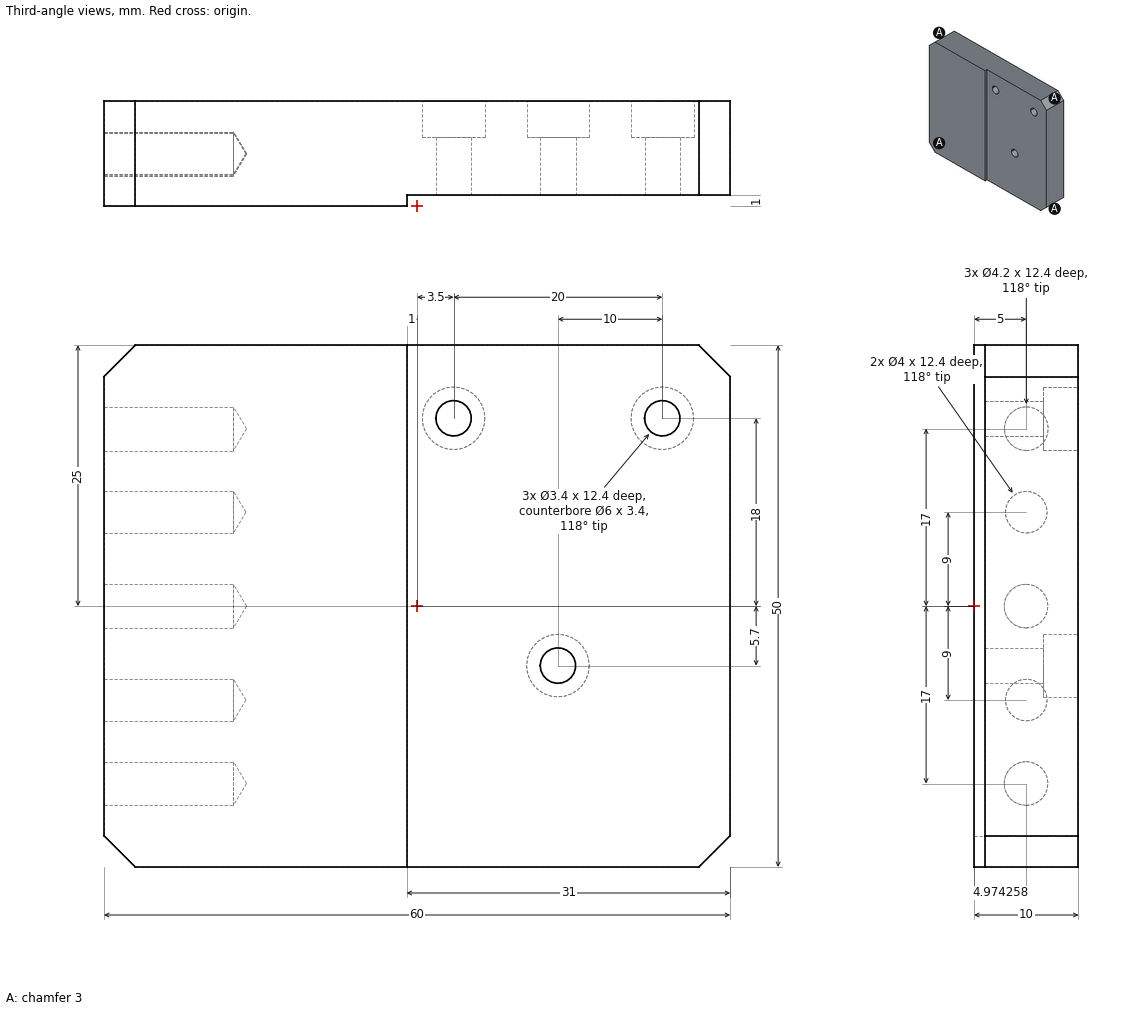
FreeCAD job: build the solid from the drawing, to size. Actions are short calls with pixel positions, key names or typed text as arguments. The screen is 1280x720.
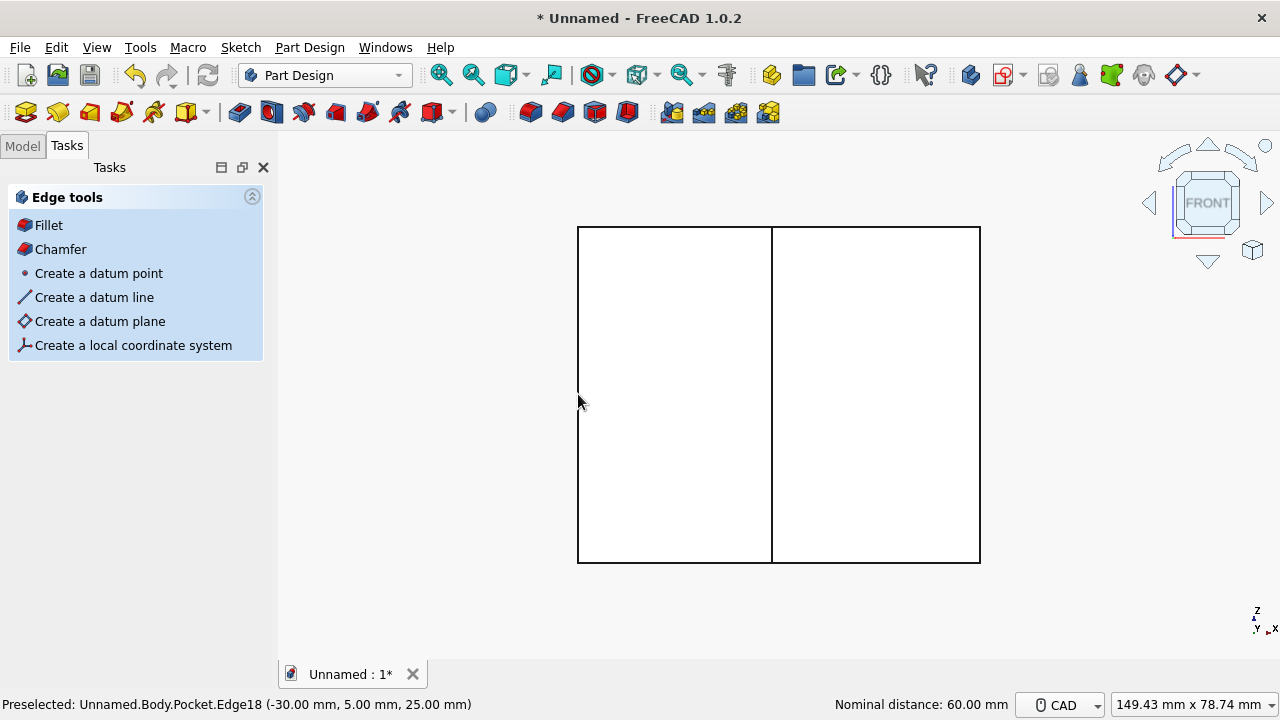
key(3)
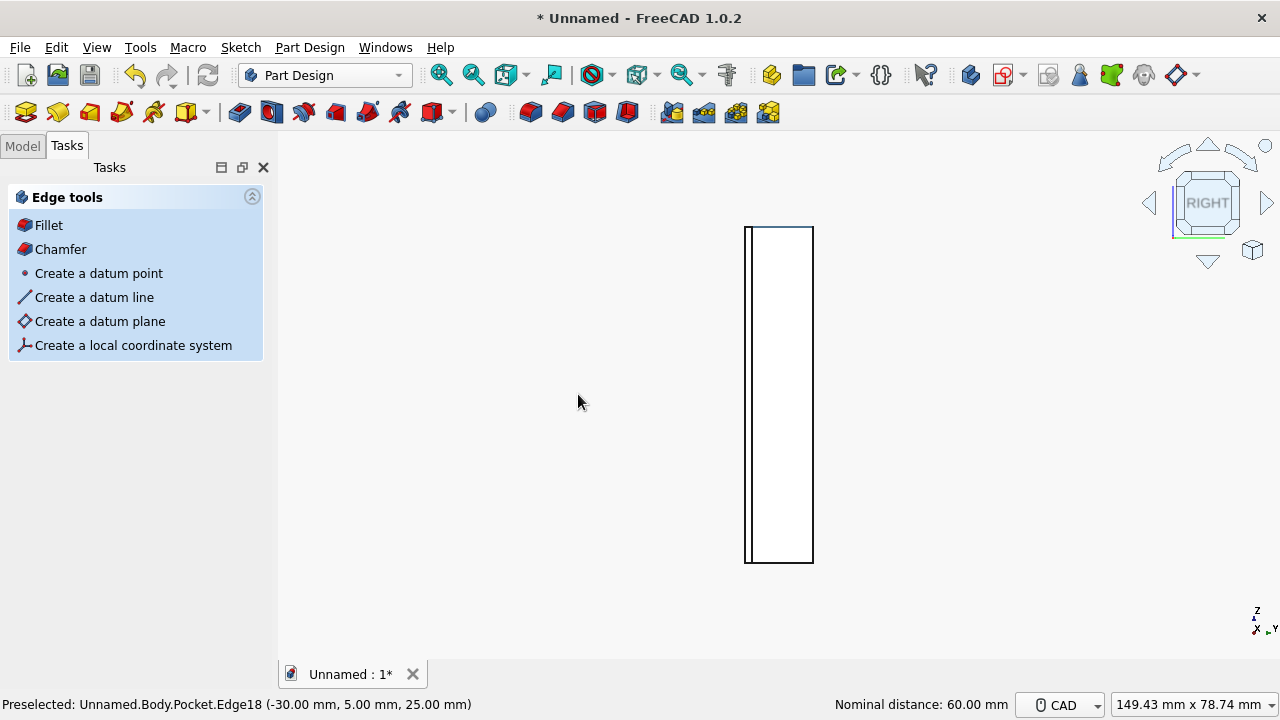
click(782, 562, ctrl)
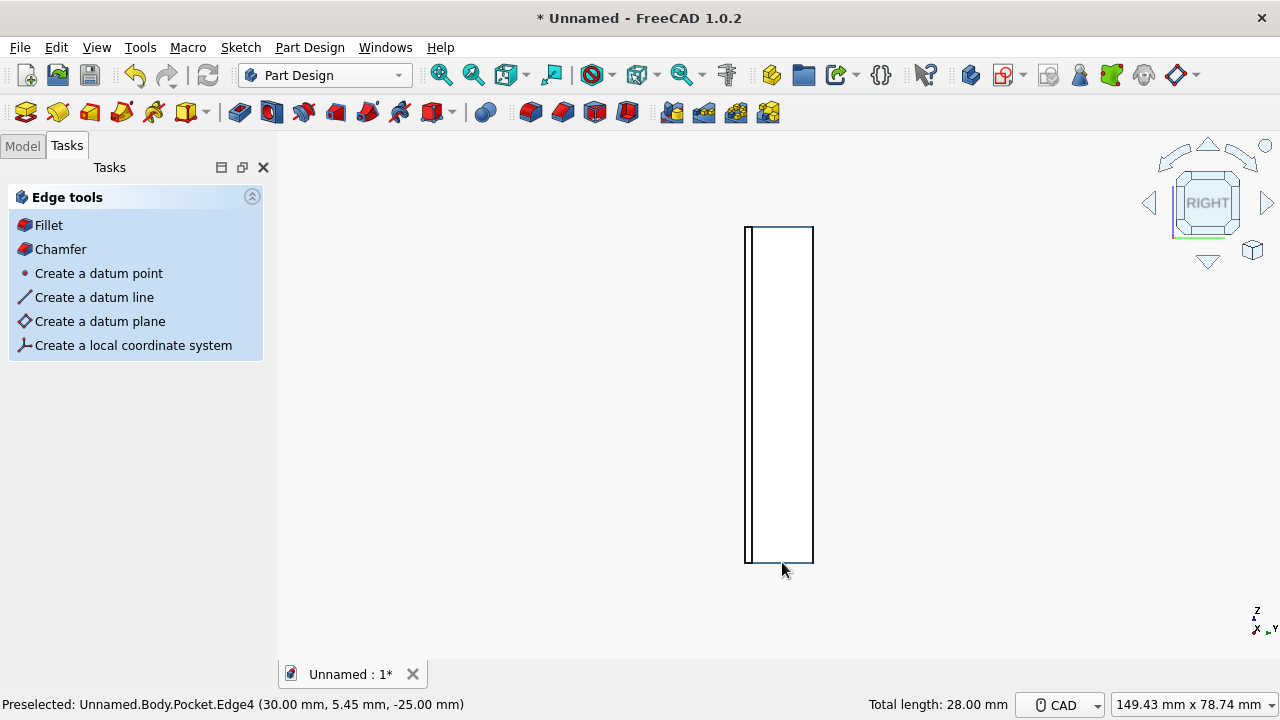
key(5)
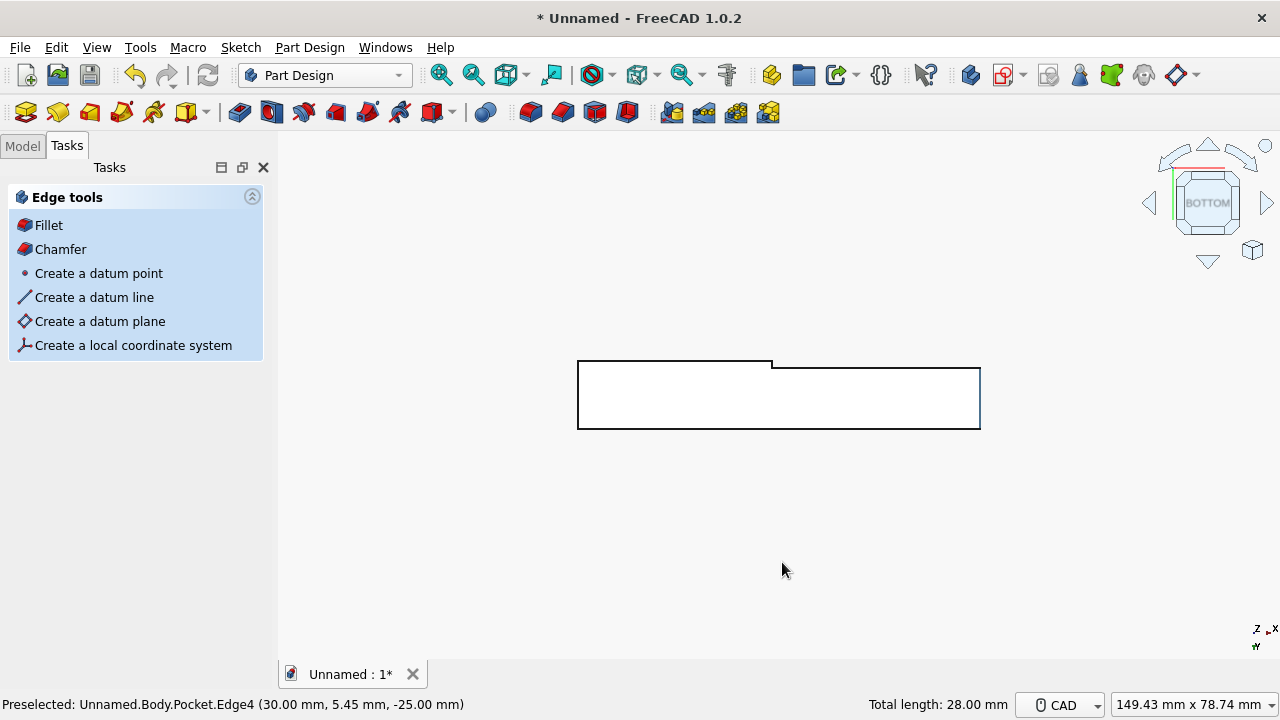
click(442, 76)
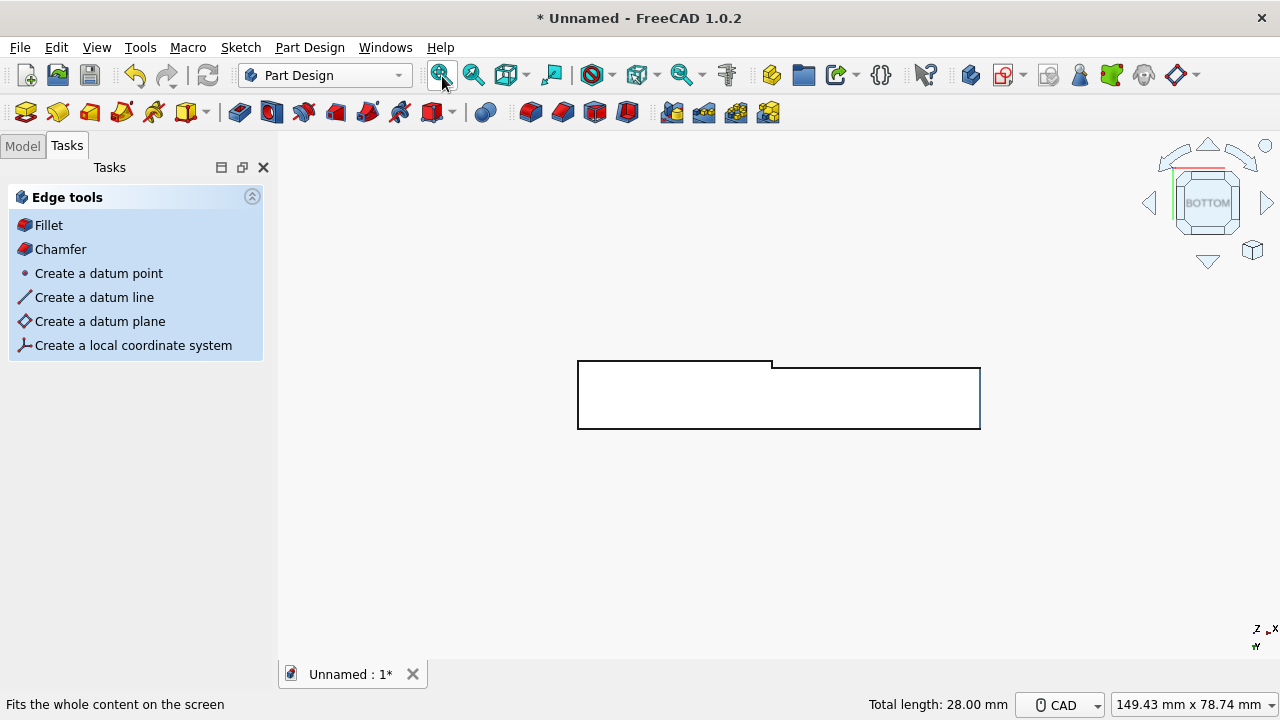
click(578, 394, ctrl)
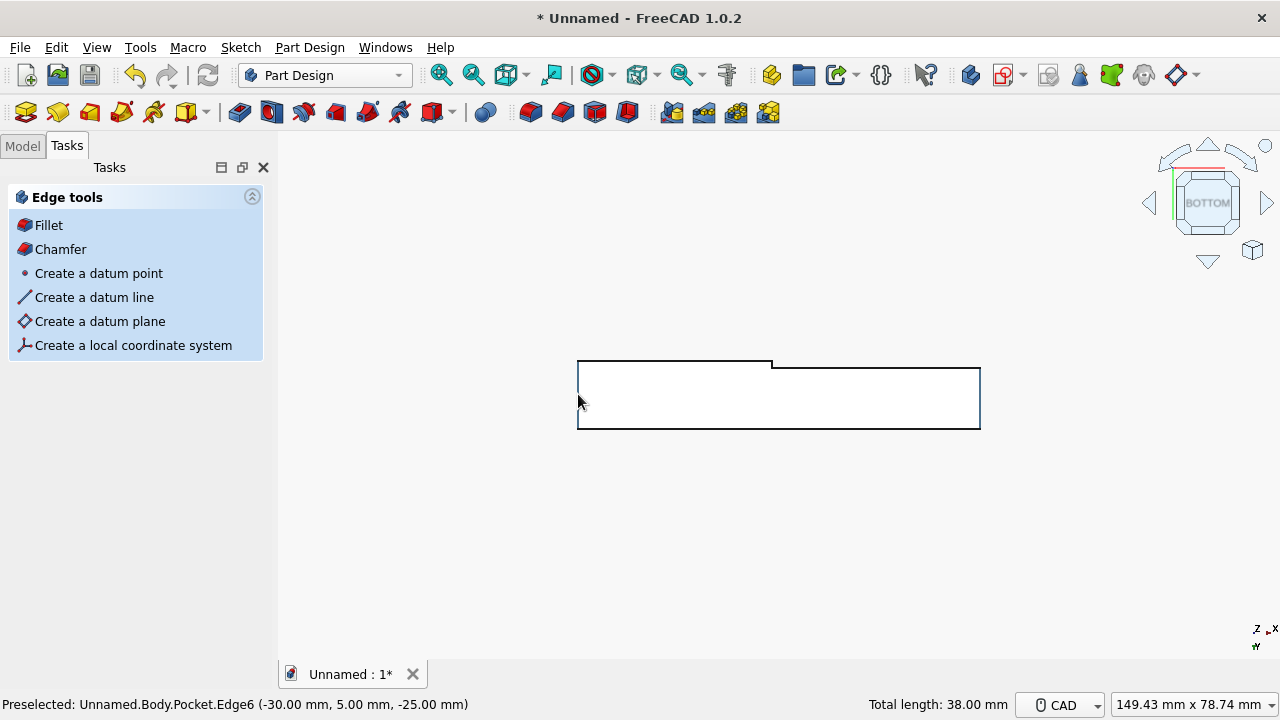
click(564, 112)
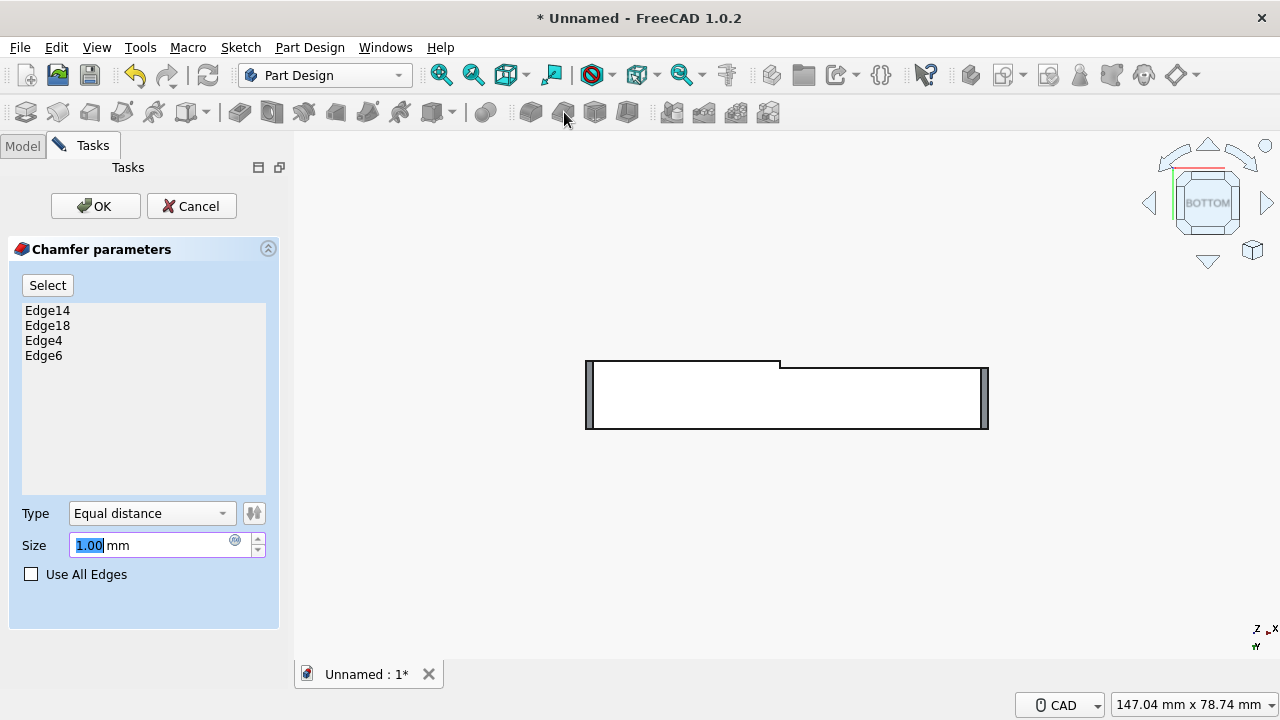
text(3)
key(Tab)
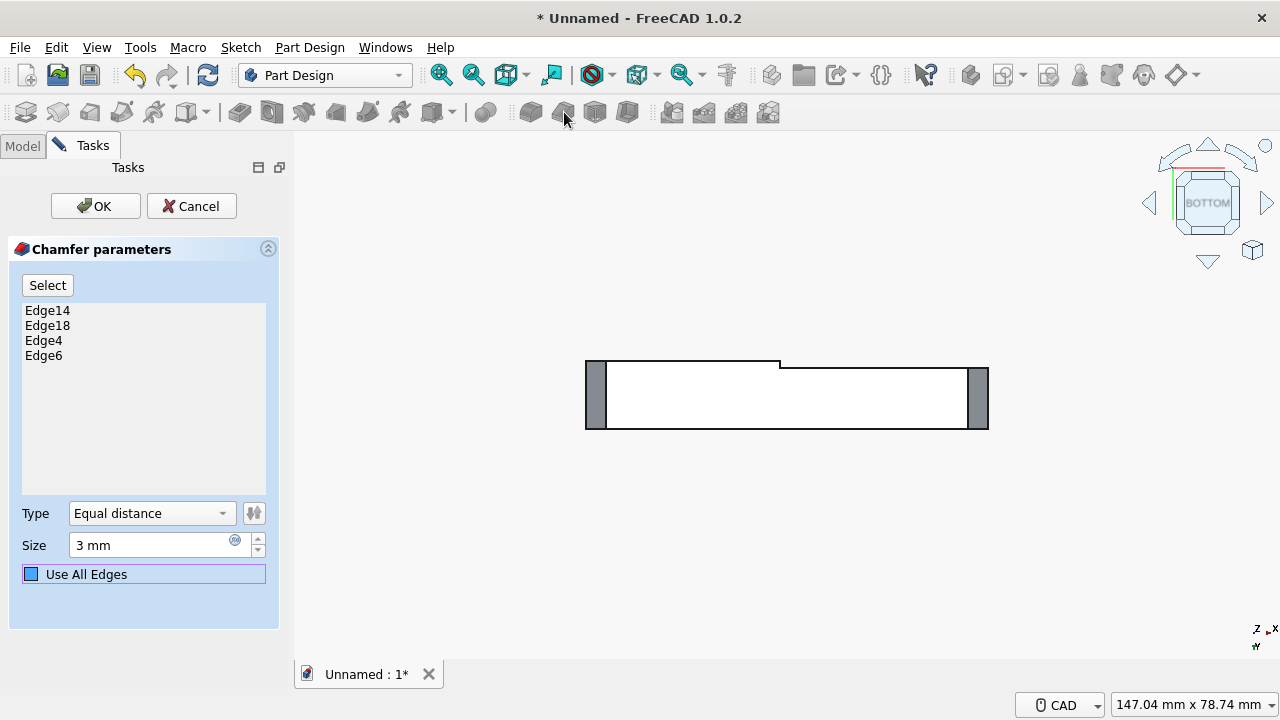
click(96, 206)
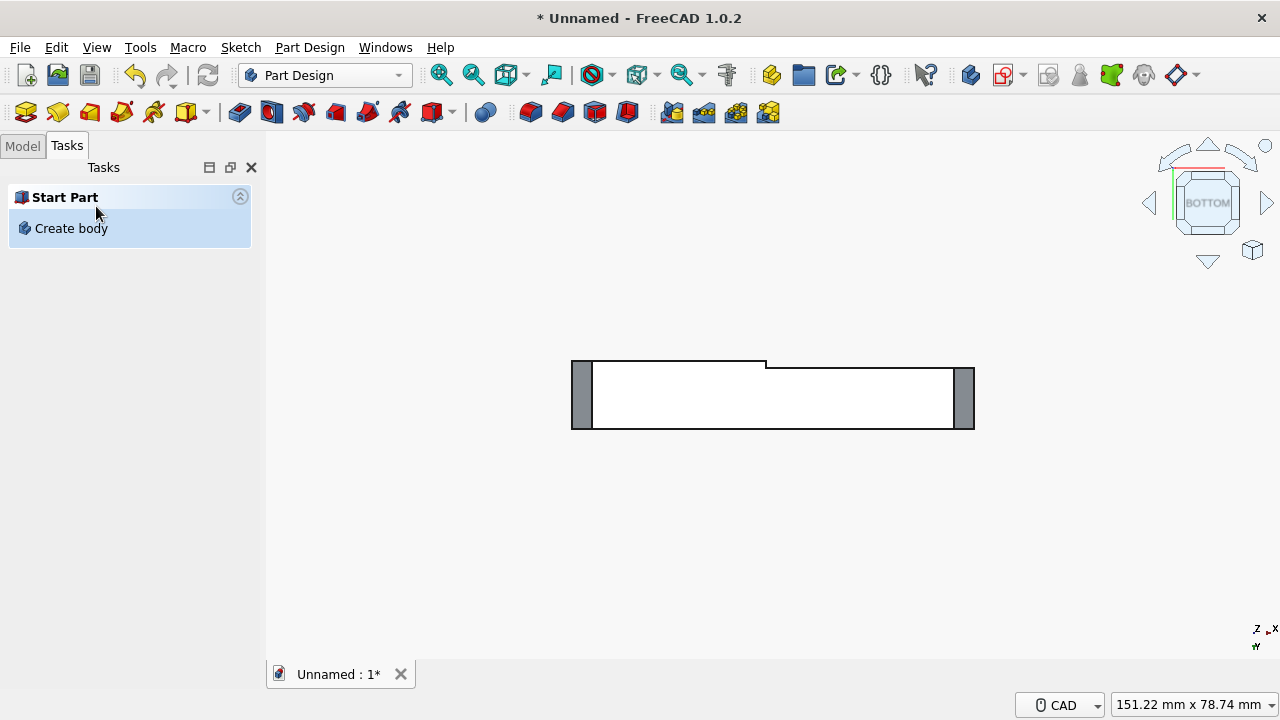
click(442, 76)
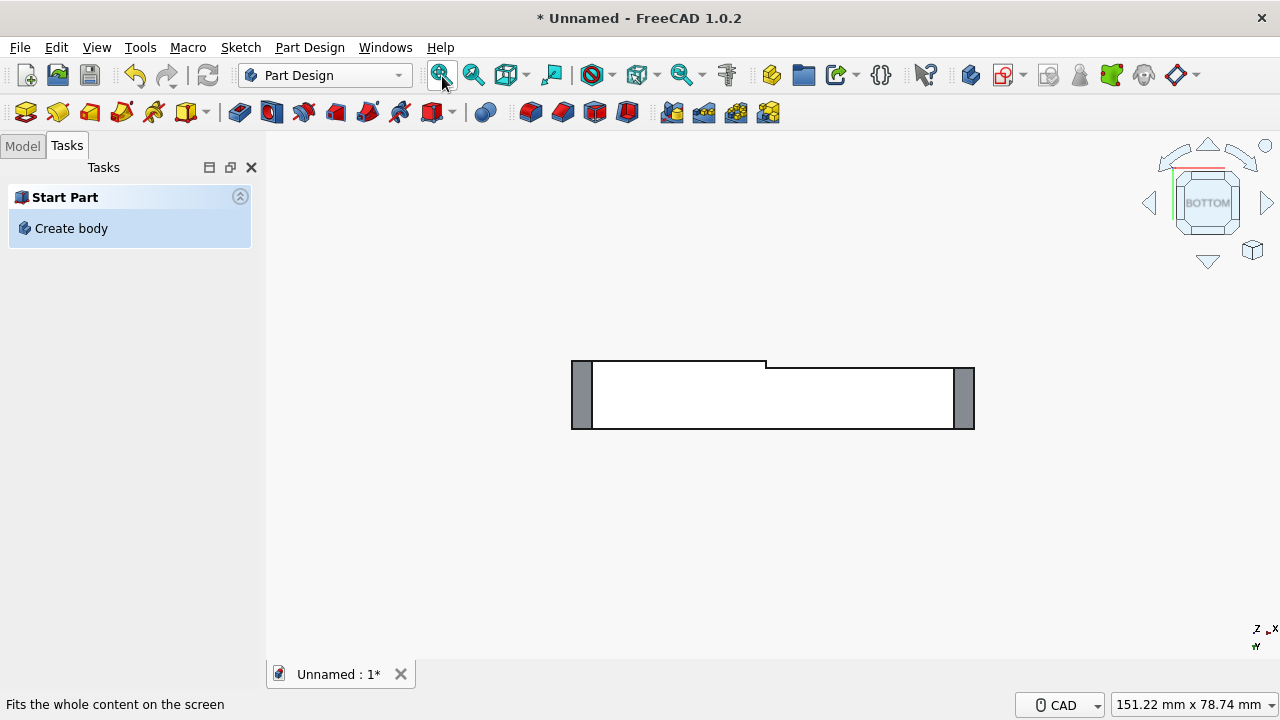
key(6)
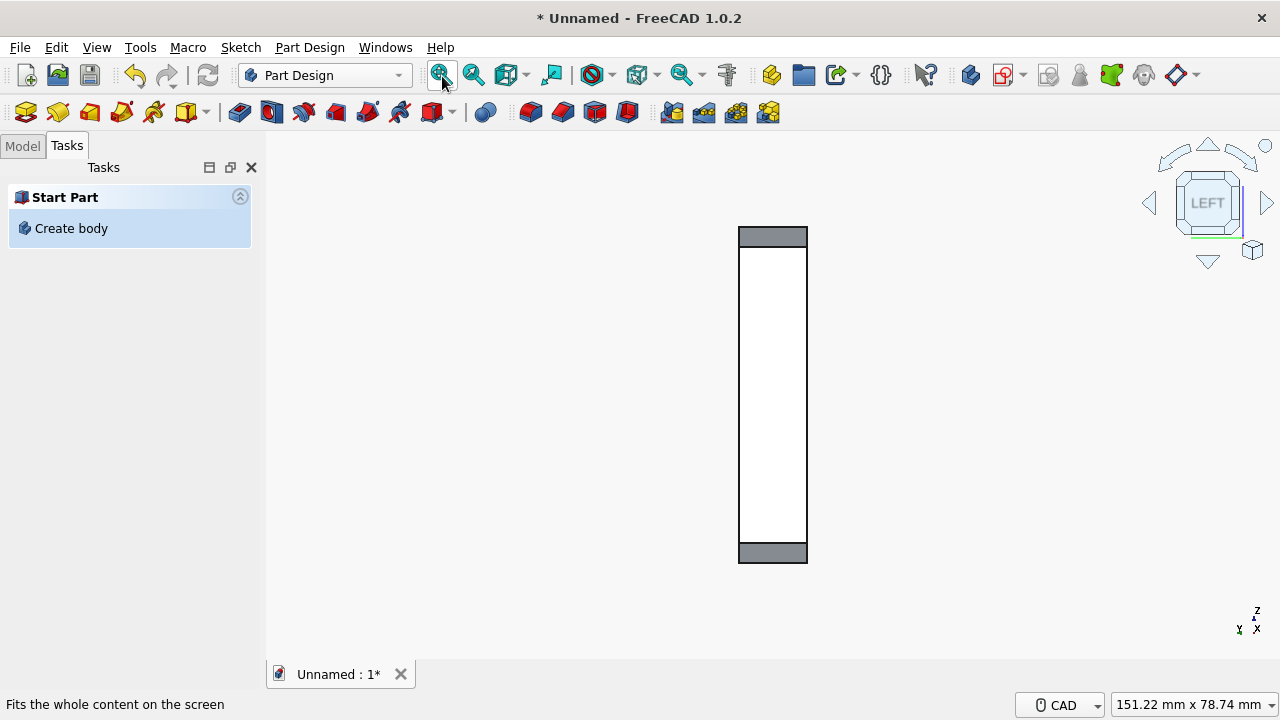
click(773, 394)